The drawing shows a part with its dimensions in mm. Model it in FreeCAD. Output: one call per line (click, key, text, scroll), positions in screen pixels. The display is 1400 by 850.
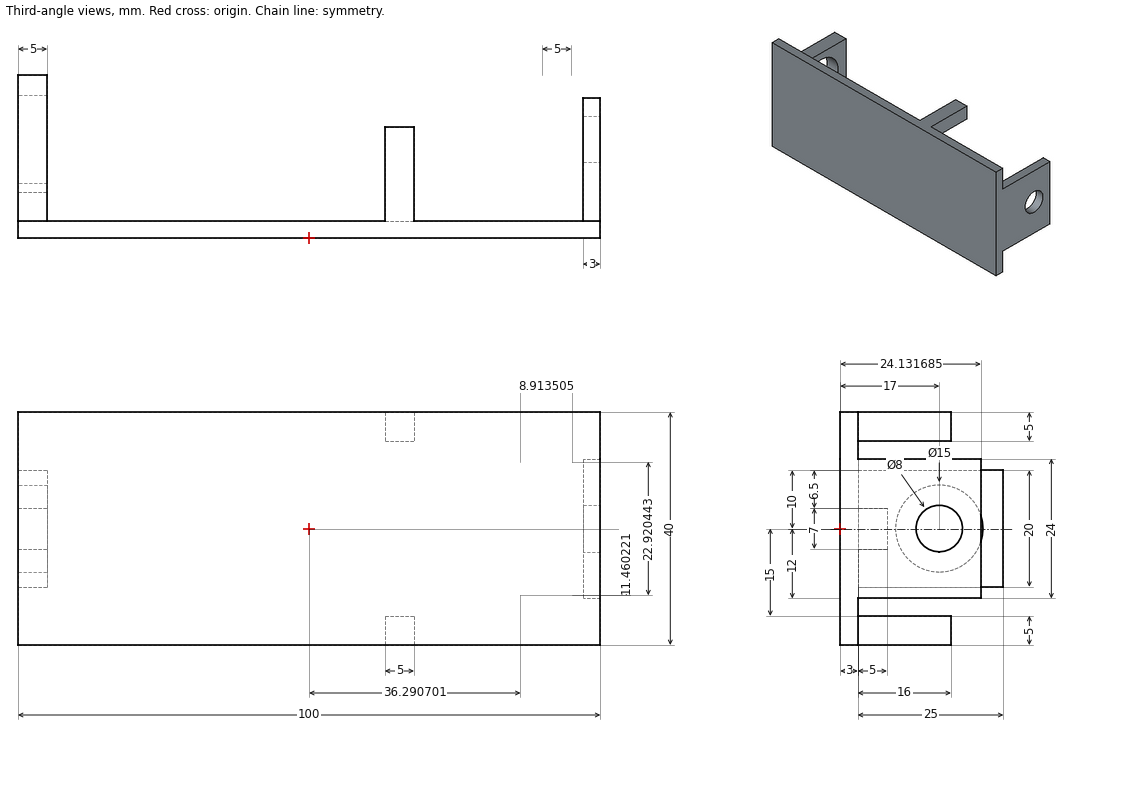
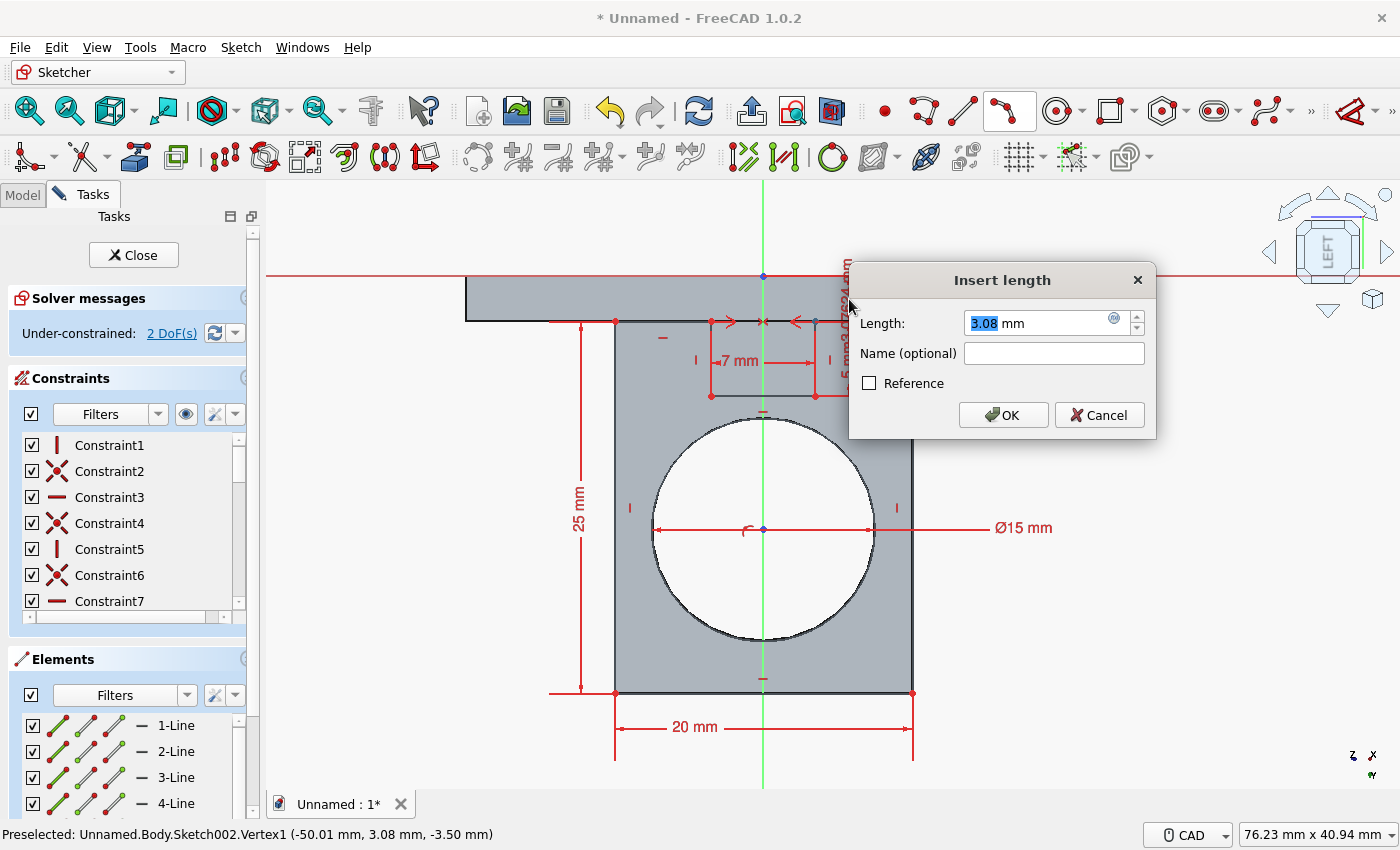
text(3)
key(Return)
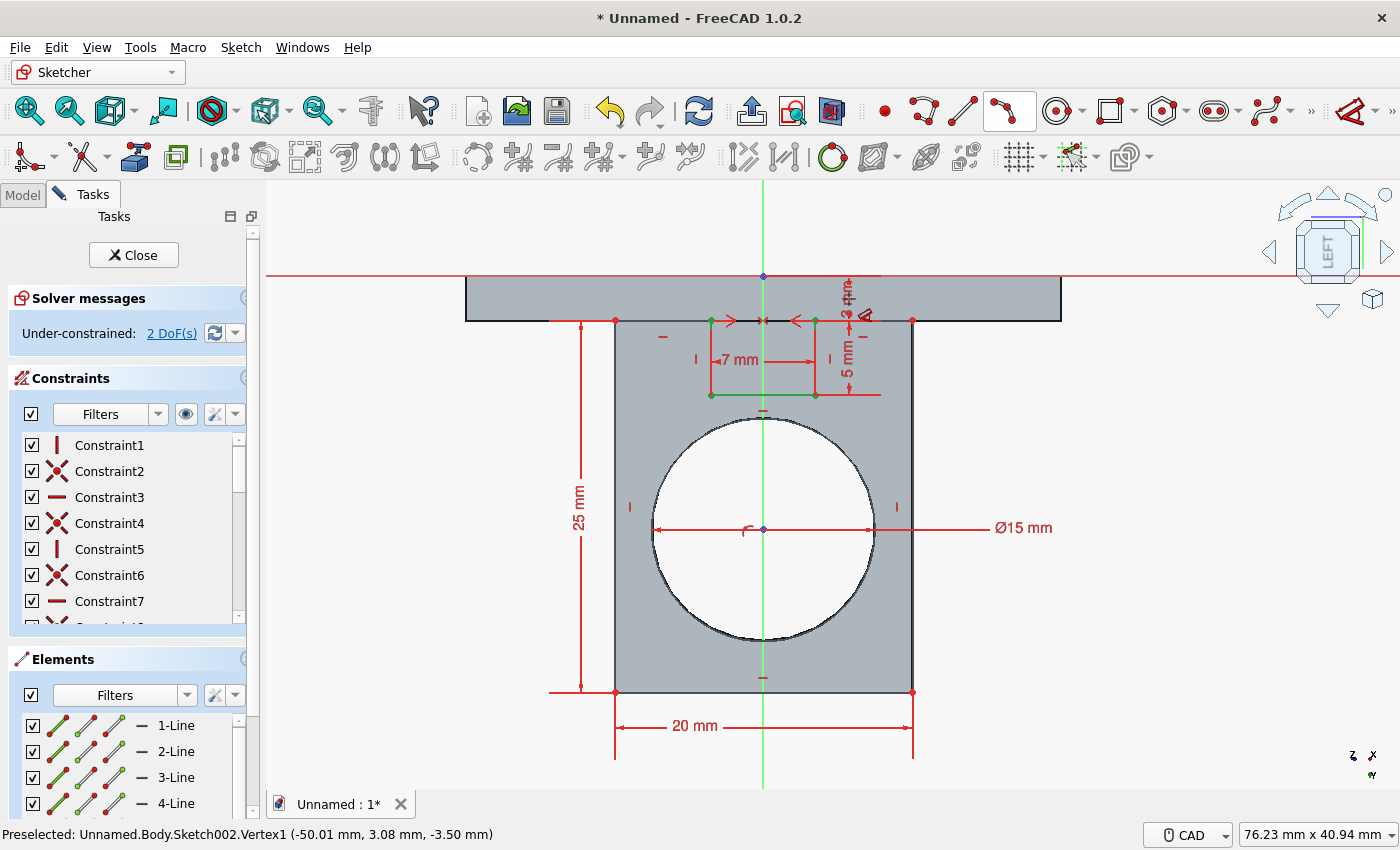
click(763, 530)
click(797, 461)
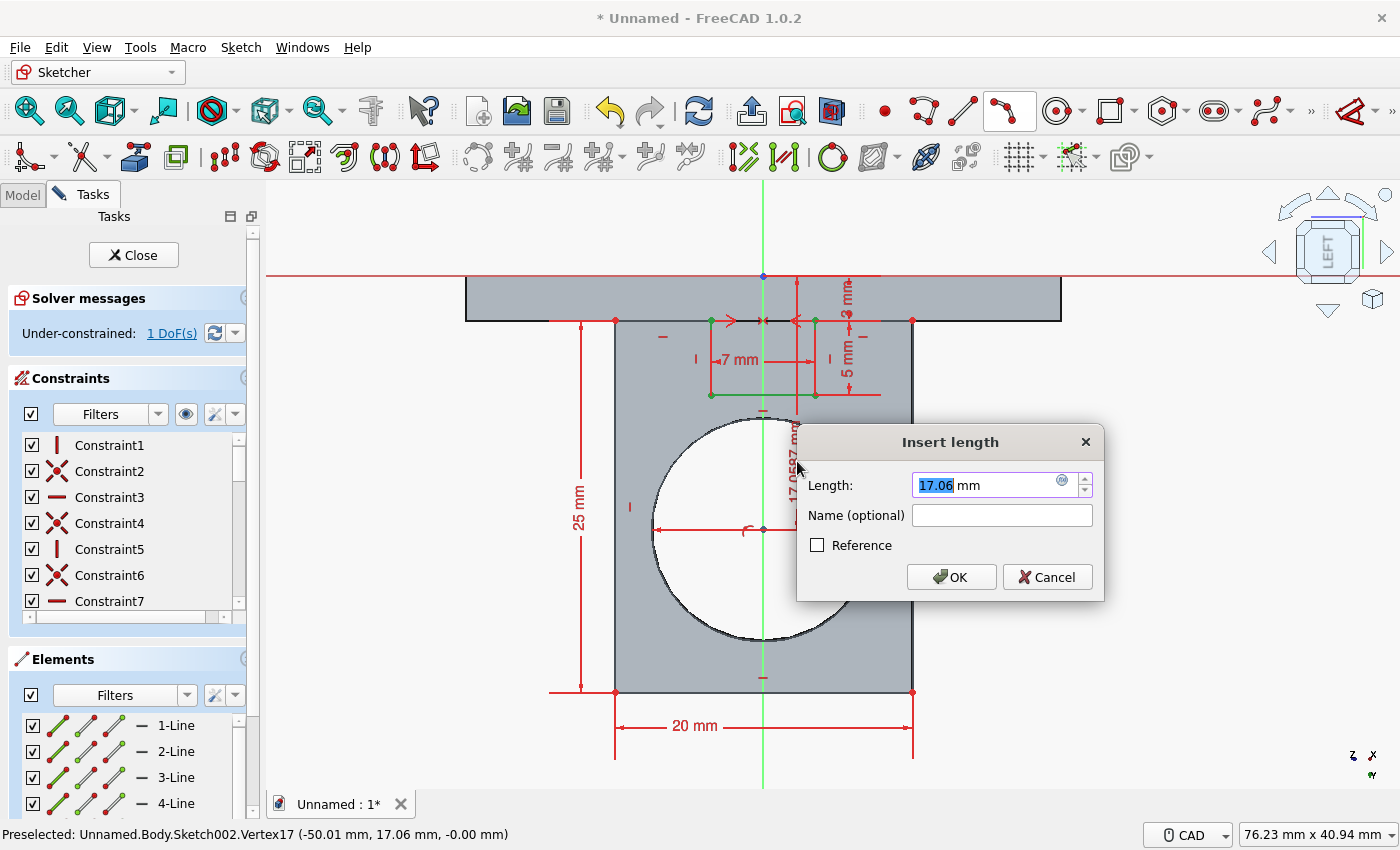
text(17)
key(Return)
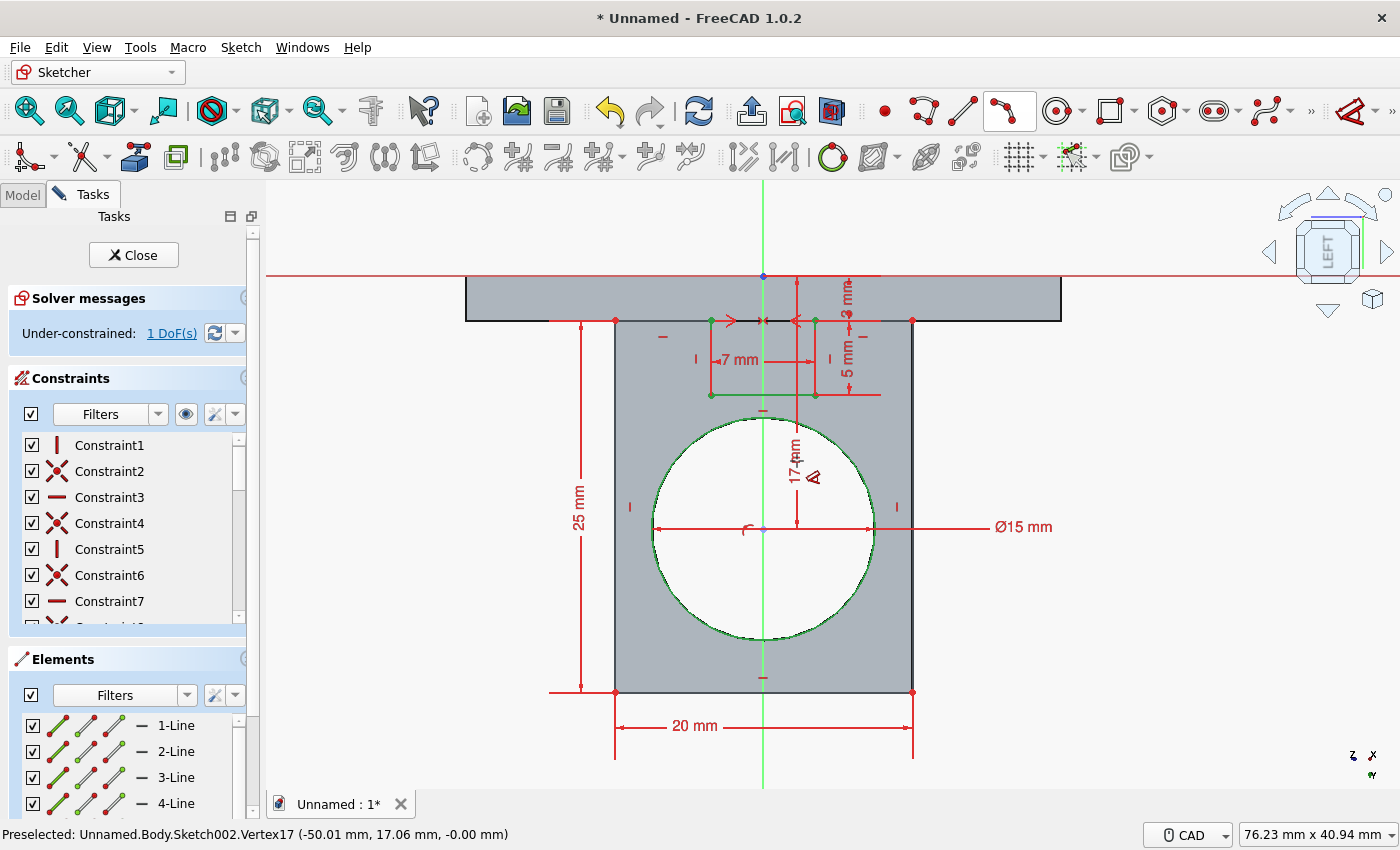
click(682, 321)
click(663, 355)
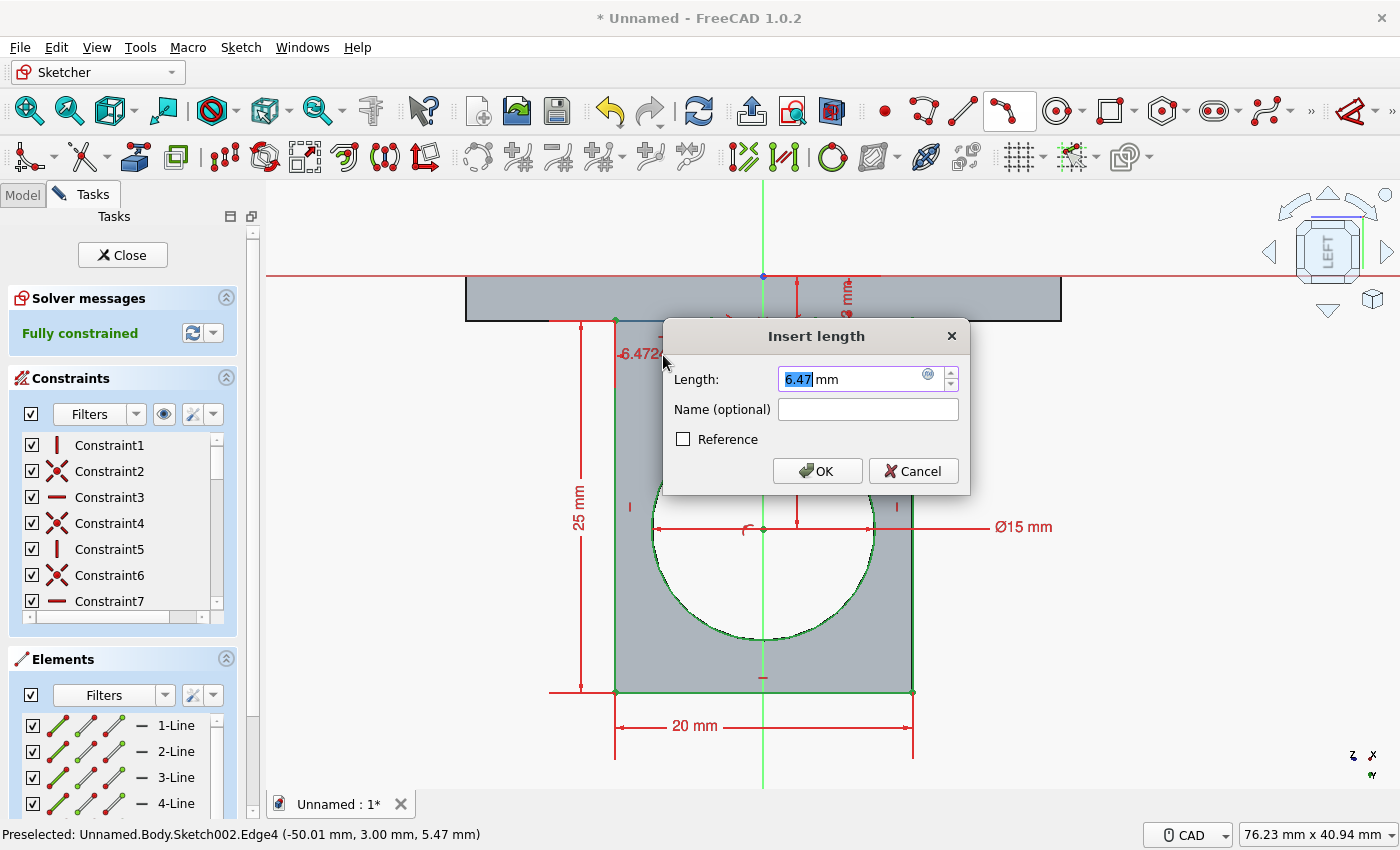
text(6.5)
key(Return)
key(Escape)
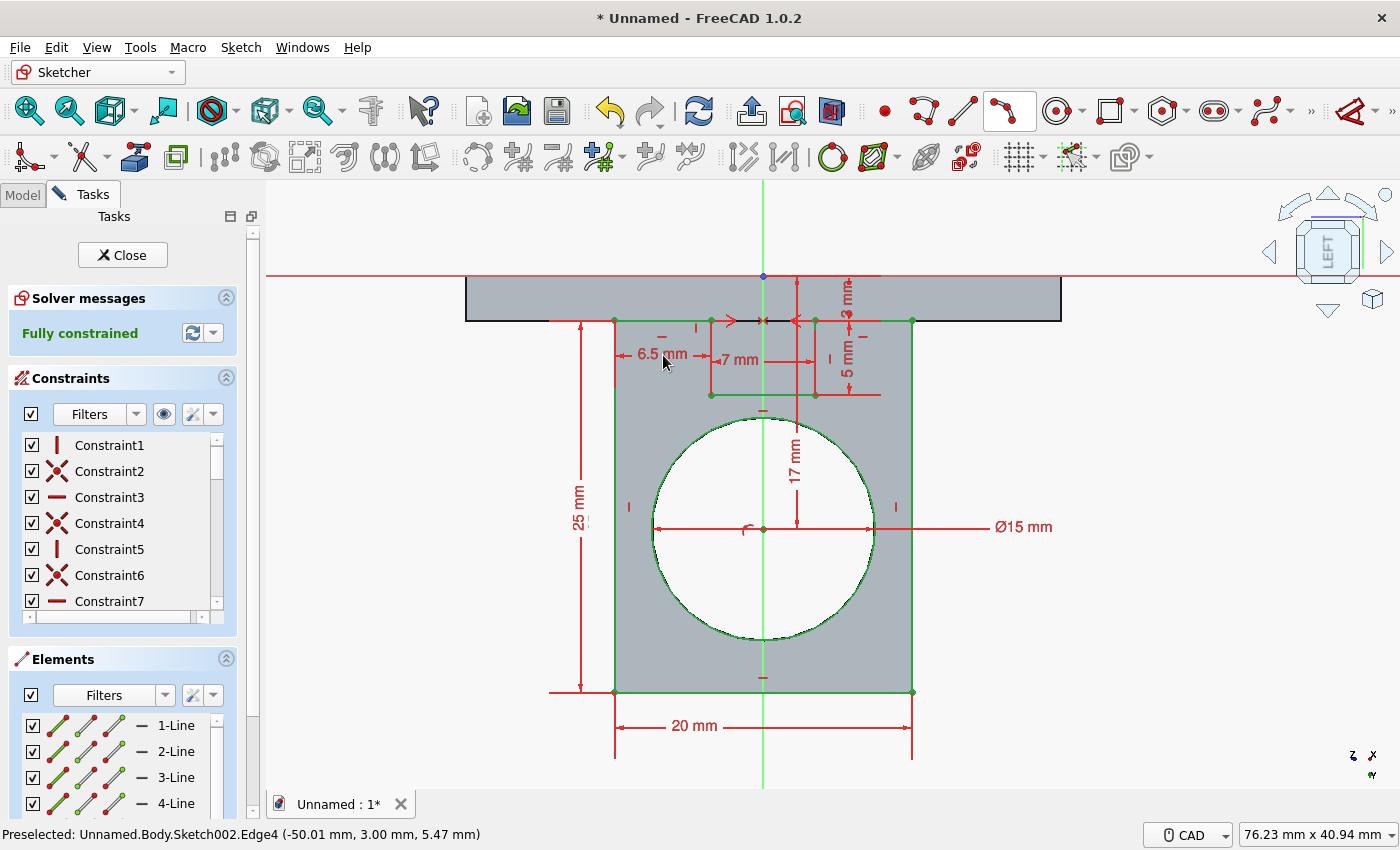
click(123, 255)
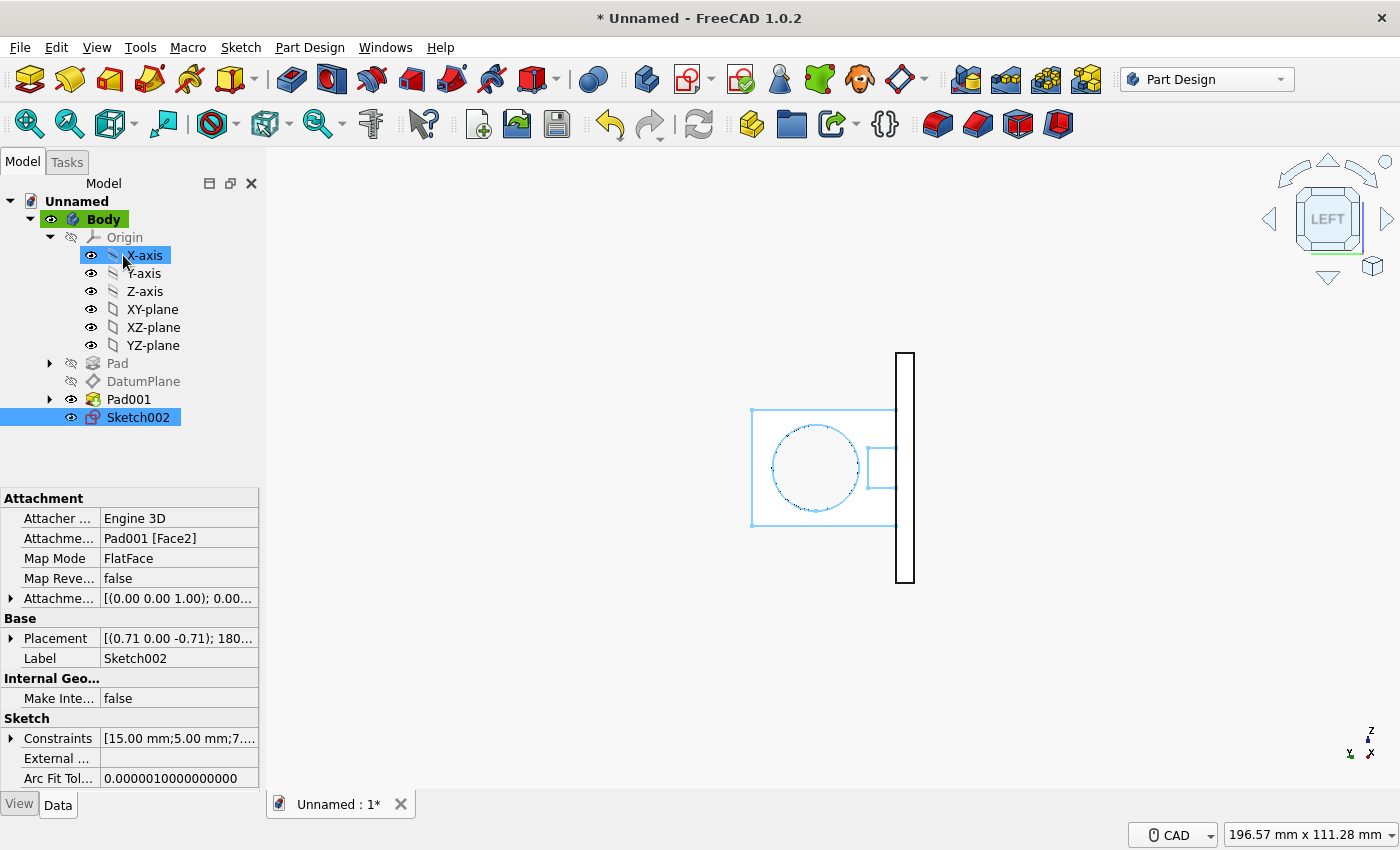
click(30, 80)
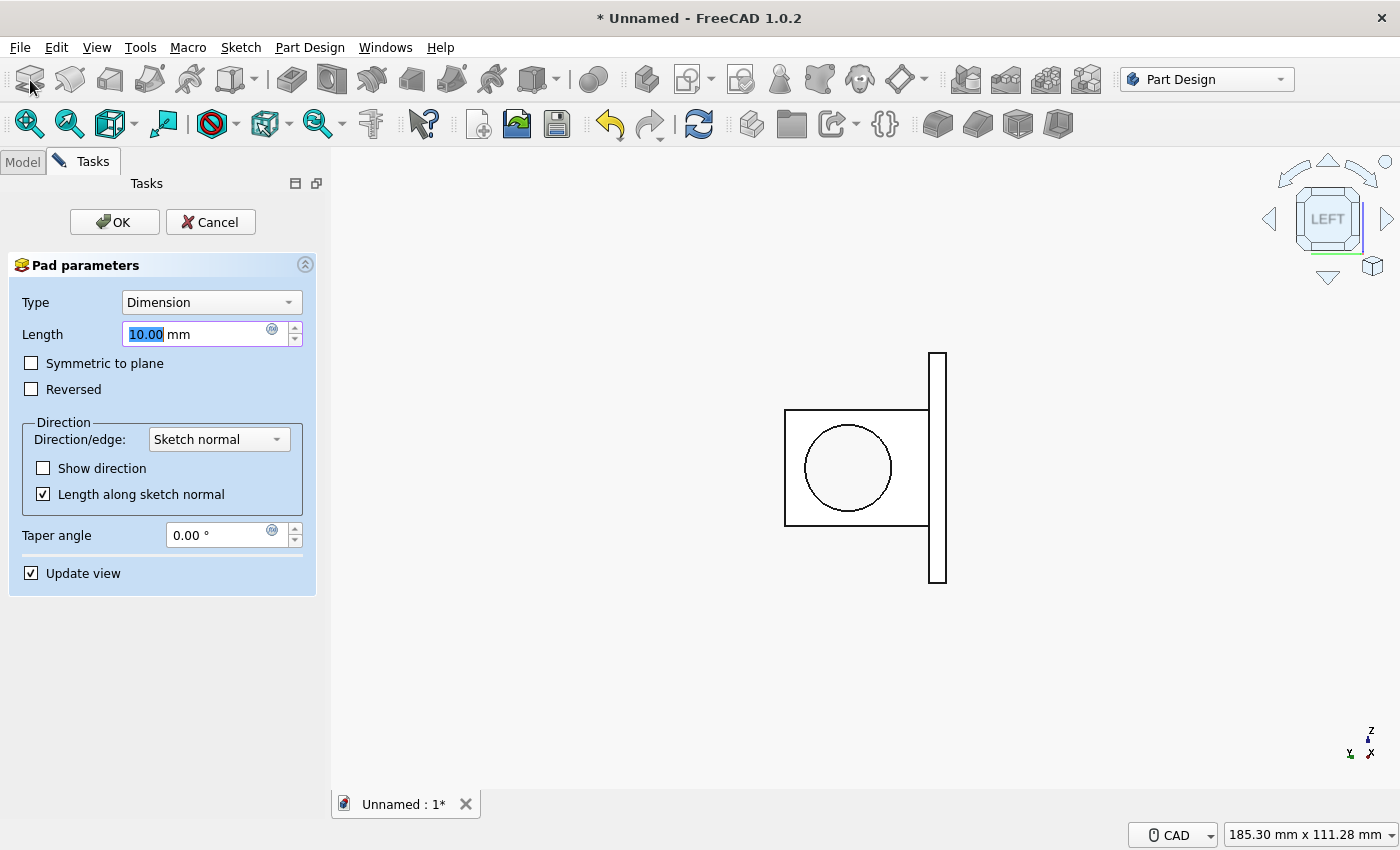
text(5)
key(Tab)